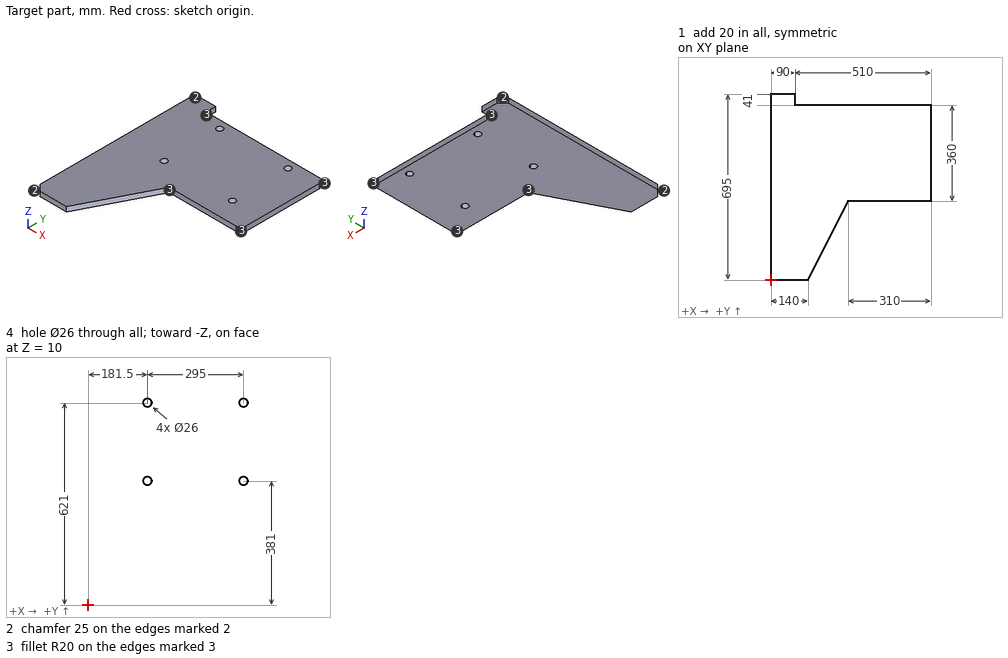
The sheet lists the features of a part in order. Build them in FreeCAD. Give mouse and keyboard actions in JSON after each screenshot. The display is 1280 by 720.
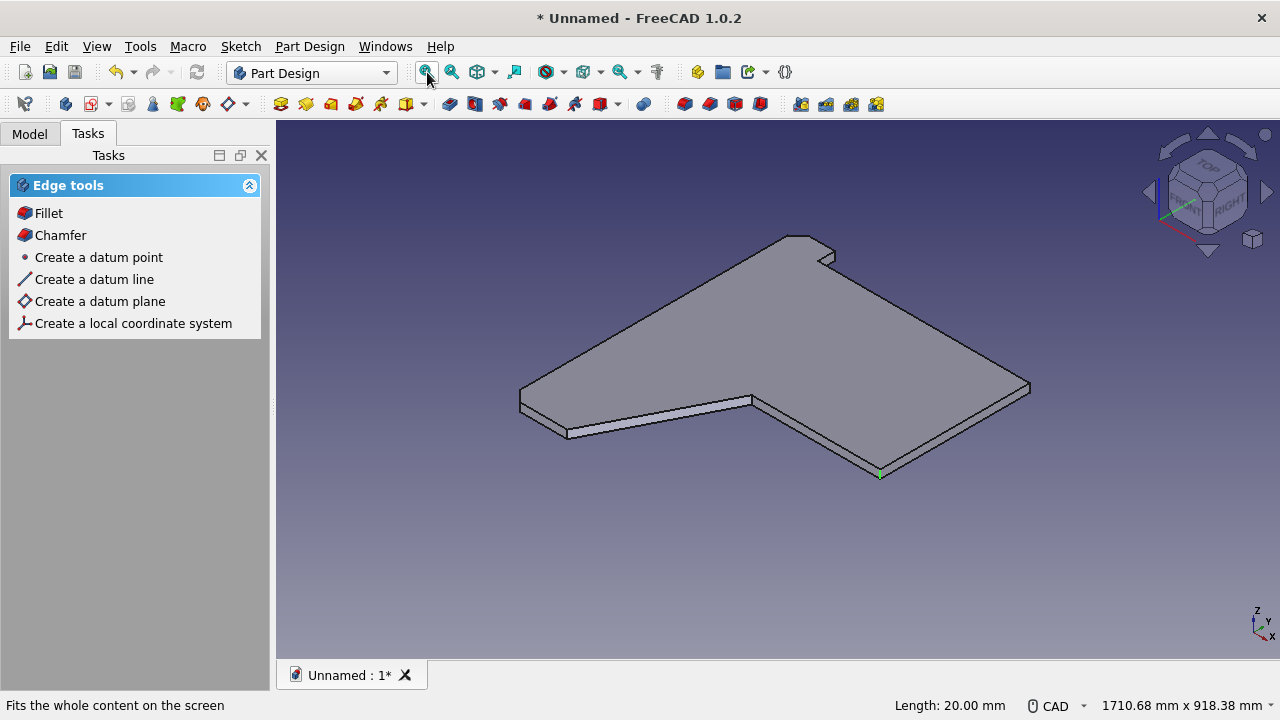
{"action": "key", "text": "2"}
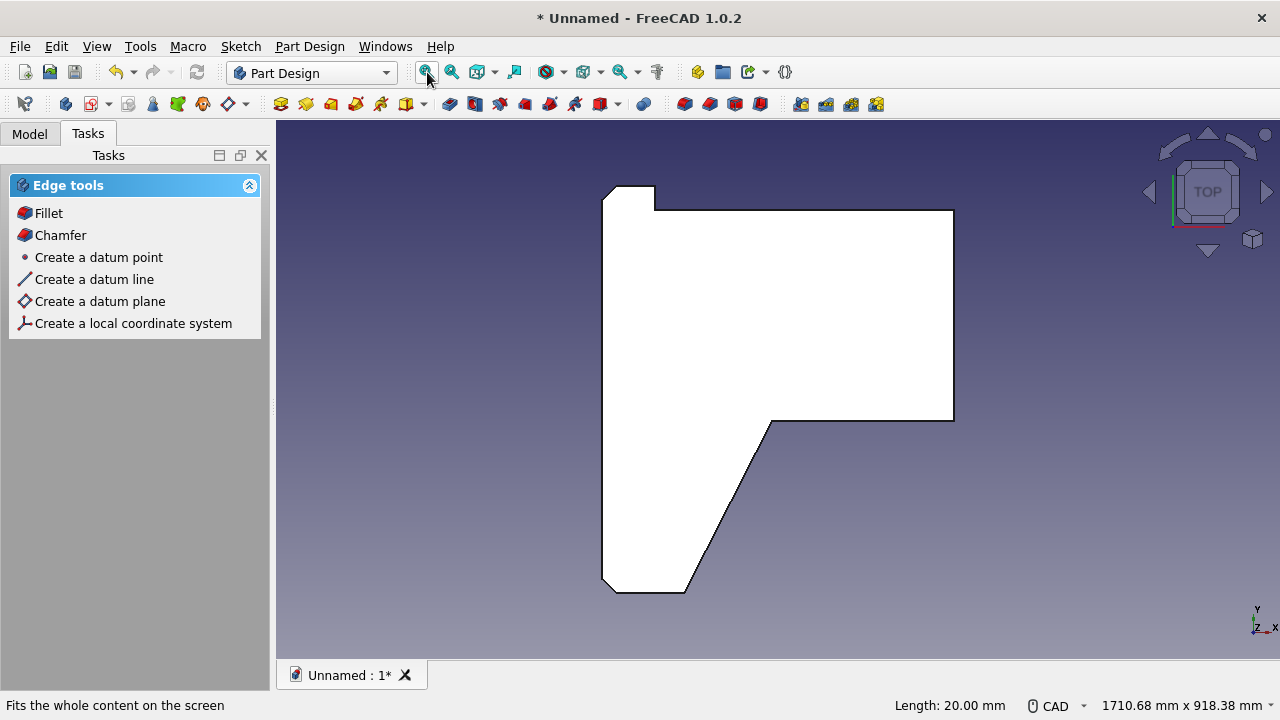
{"action": "scroll", "coordinate": [655, 209], "scroll_direction": "up", "scroll_amount": 7}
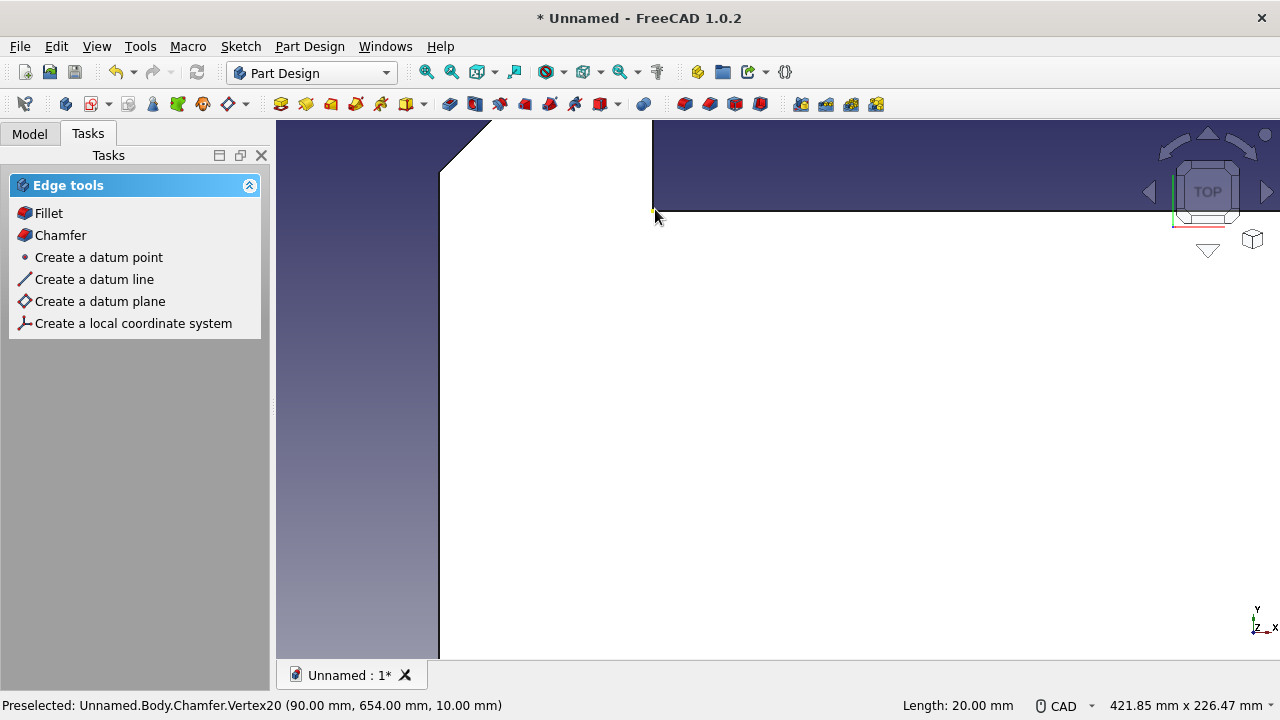
{"action": "left_click", "coordinate": [427, 72]}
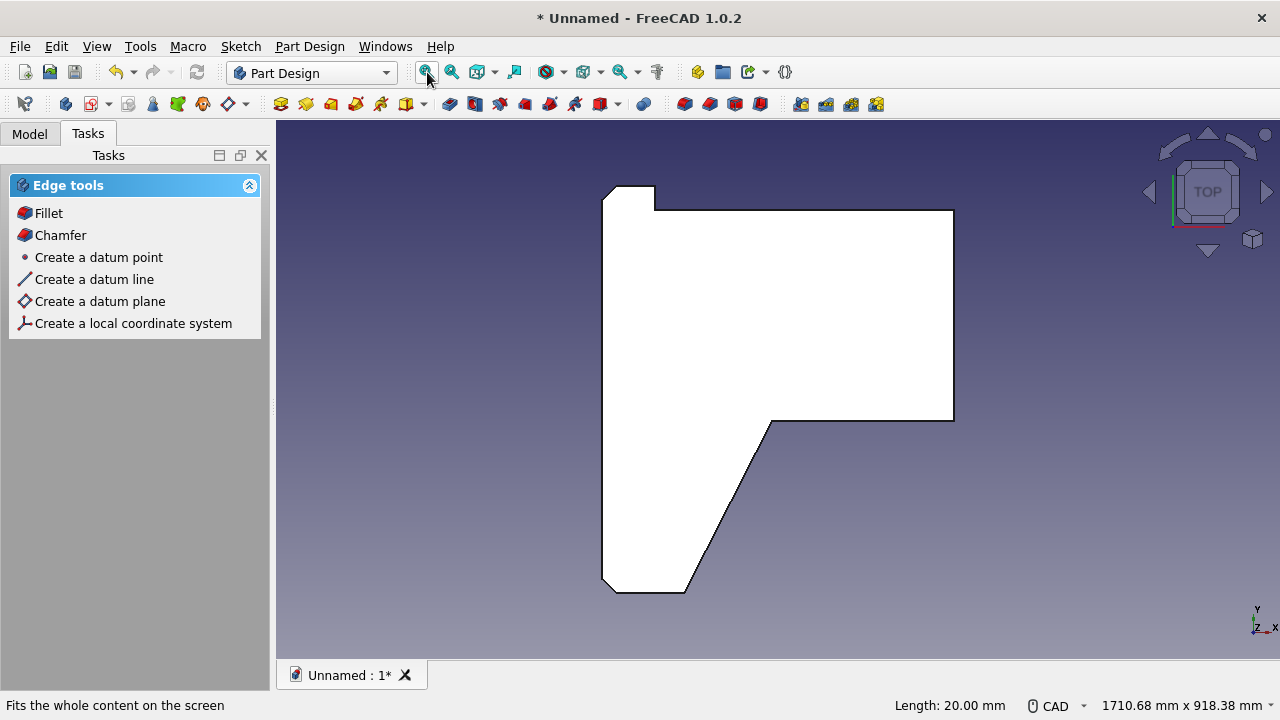
{"action": "key", "text": "1"}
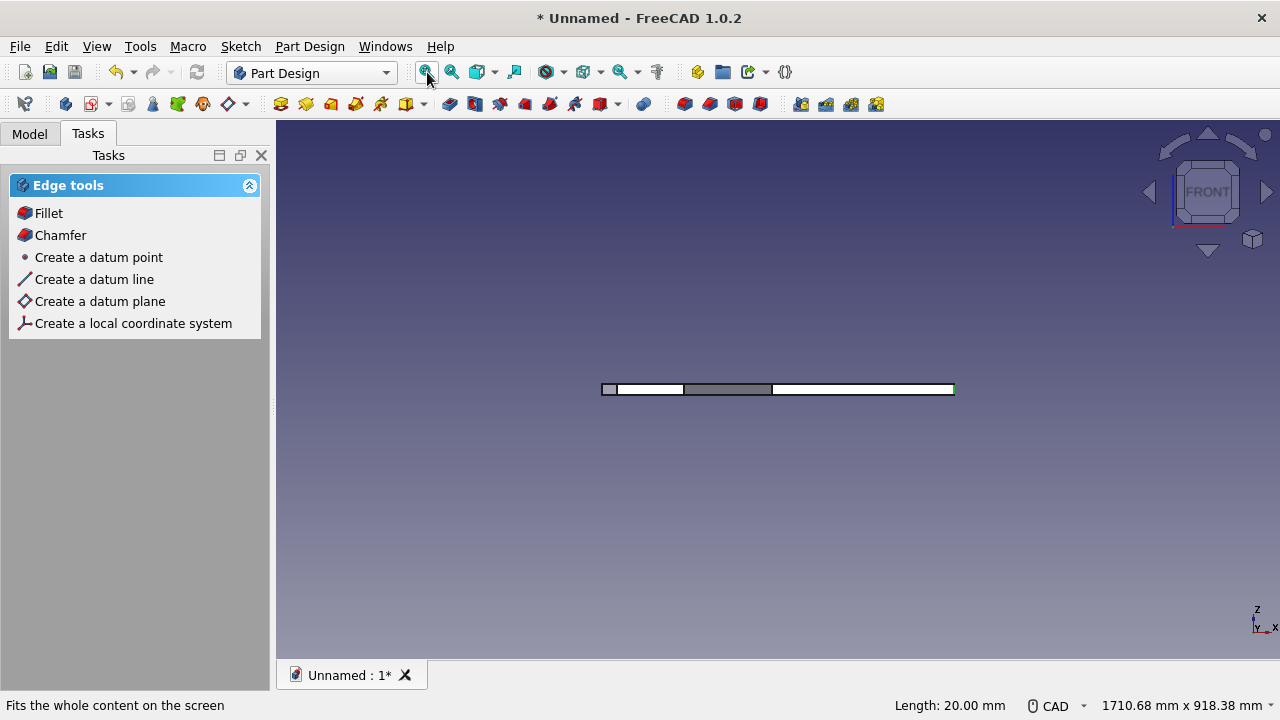
{"action": "left_click", "coordinate": [427, 72]}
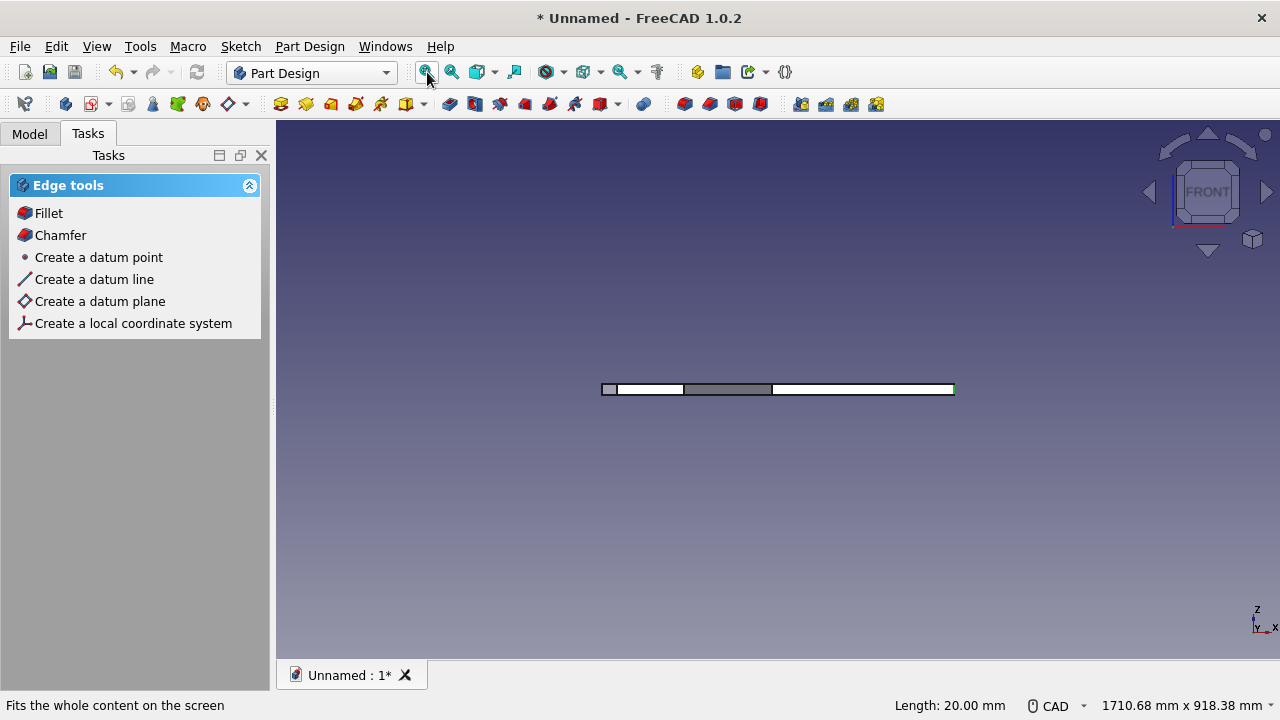
{"action": "scroll", "coordinate": [655, 389], "scroll_direction": "up", "scroll_amount": 7}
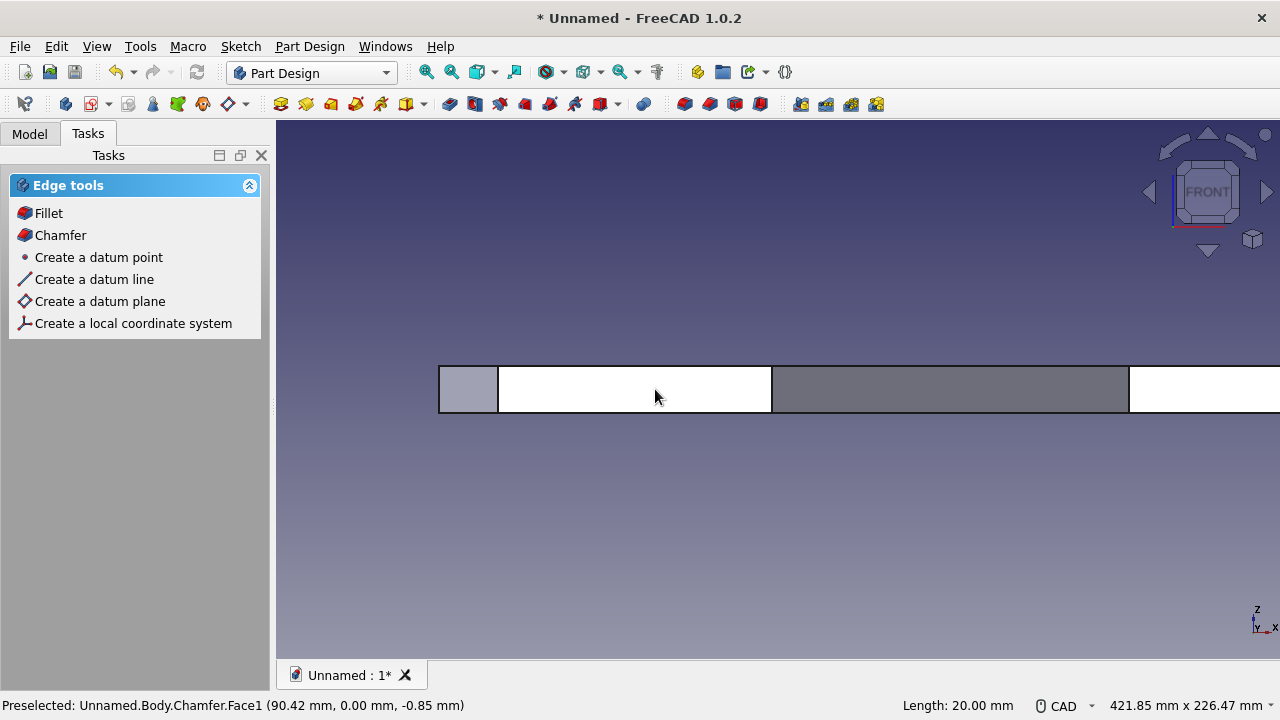
{"action": "left_click", "coordinate": [427, 72]}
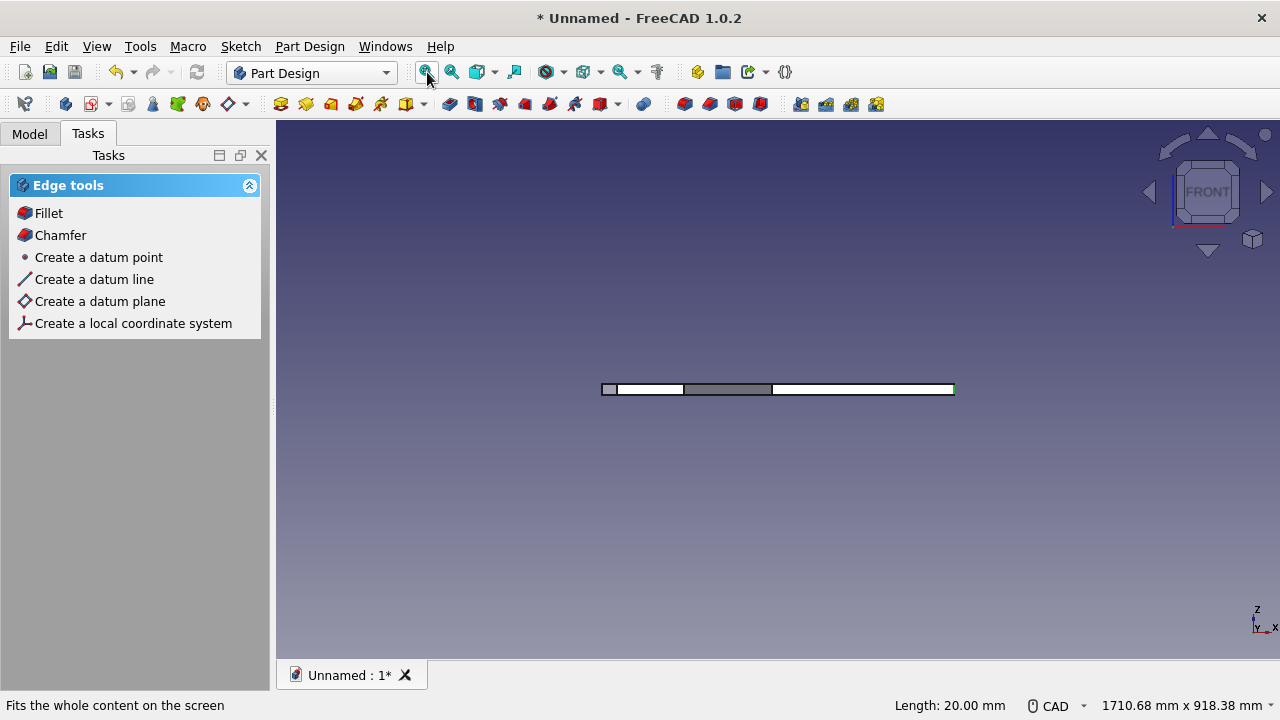
{"action": "key", "text": "3"}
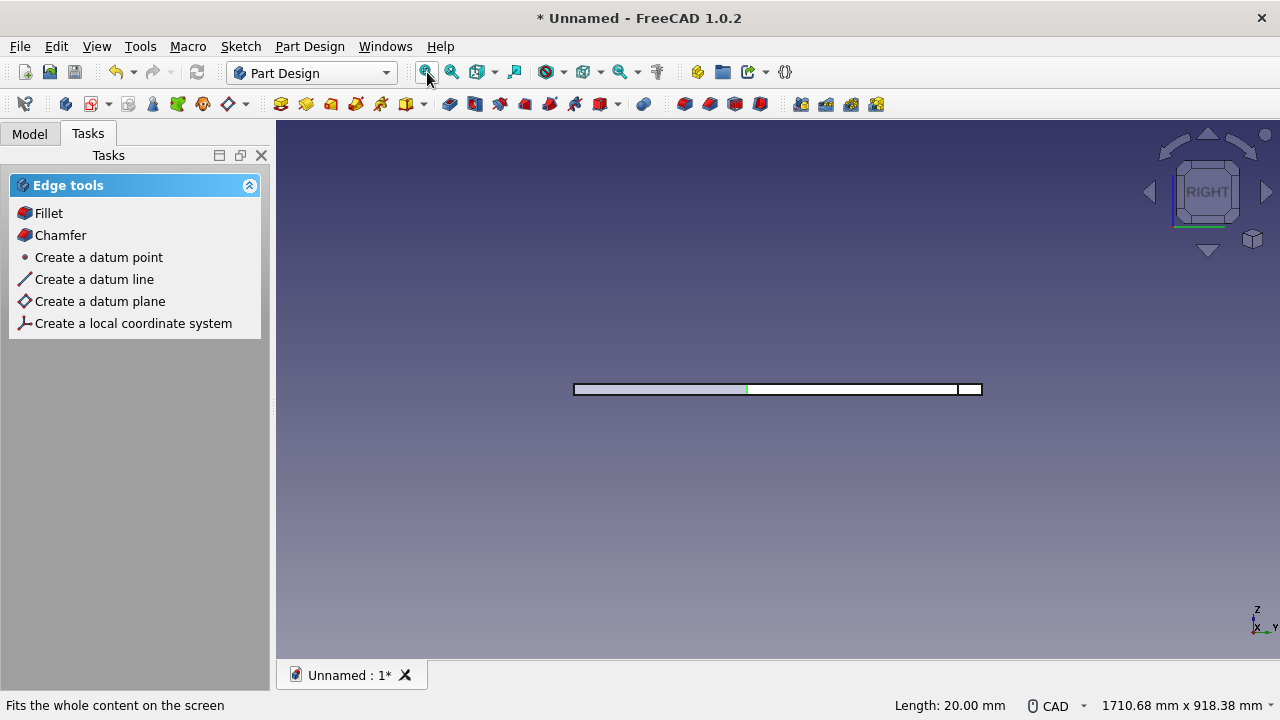
{"action": "left_click", "coordinate": [427, 72]}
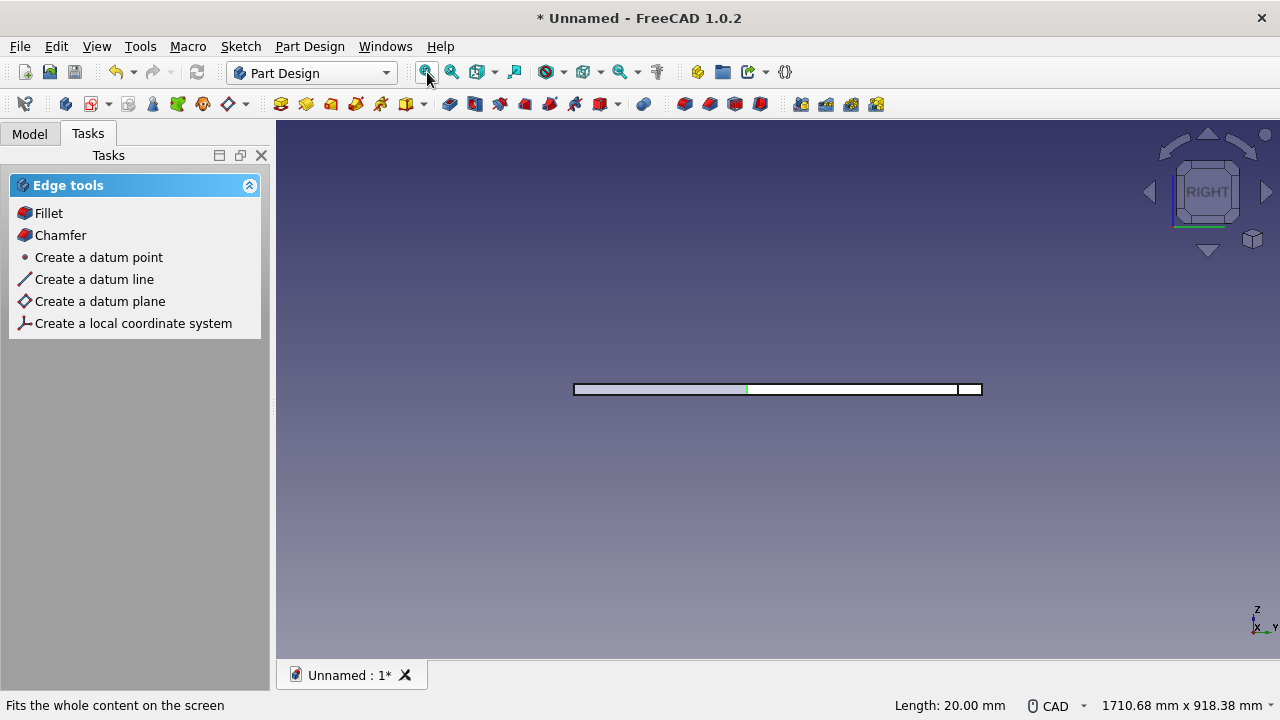
{"action": "scroll", "coordinate": [958, 388], "scroll_direction": "up", "scroll_amount": 7}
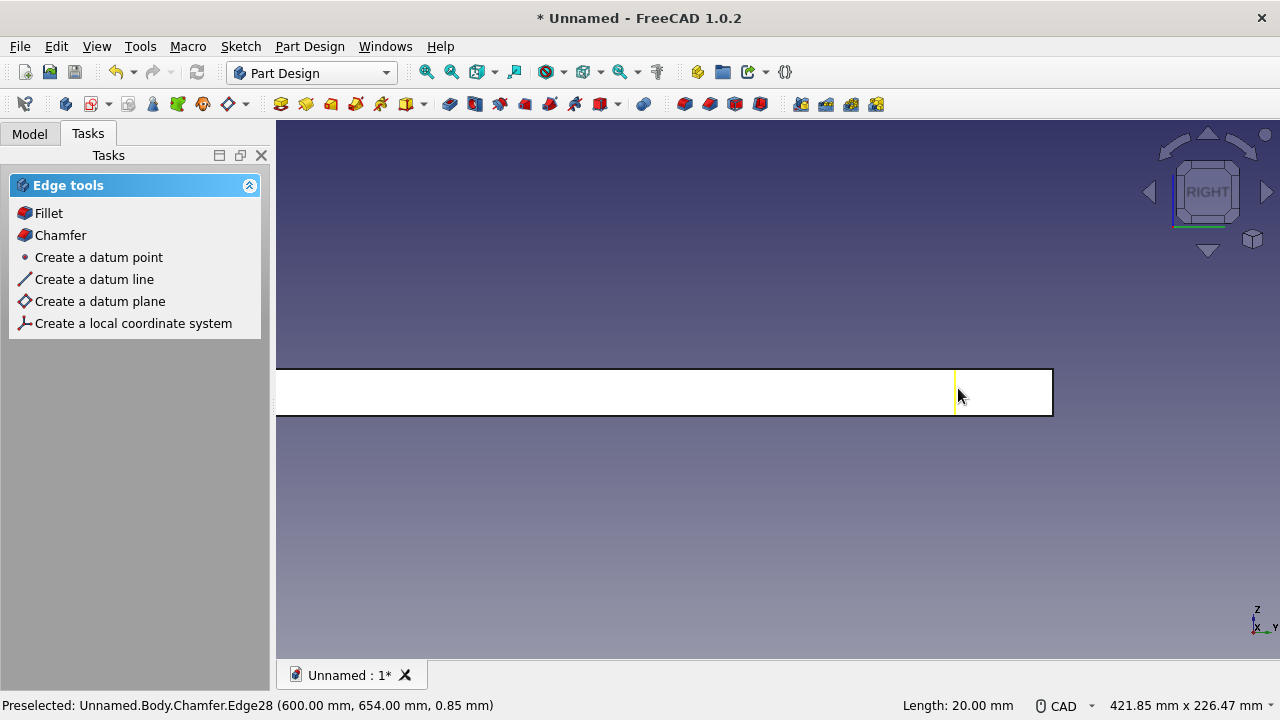
{"action": "left_click", "coordinate": [955, 392], "text": "ctrl"}